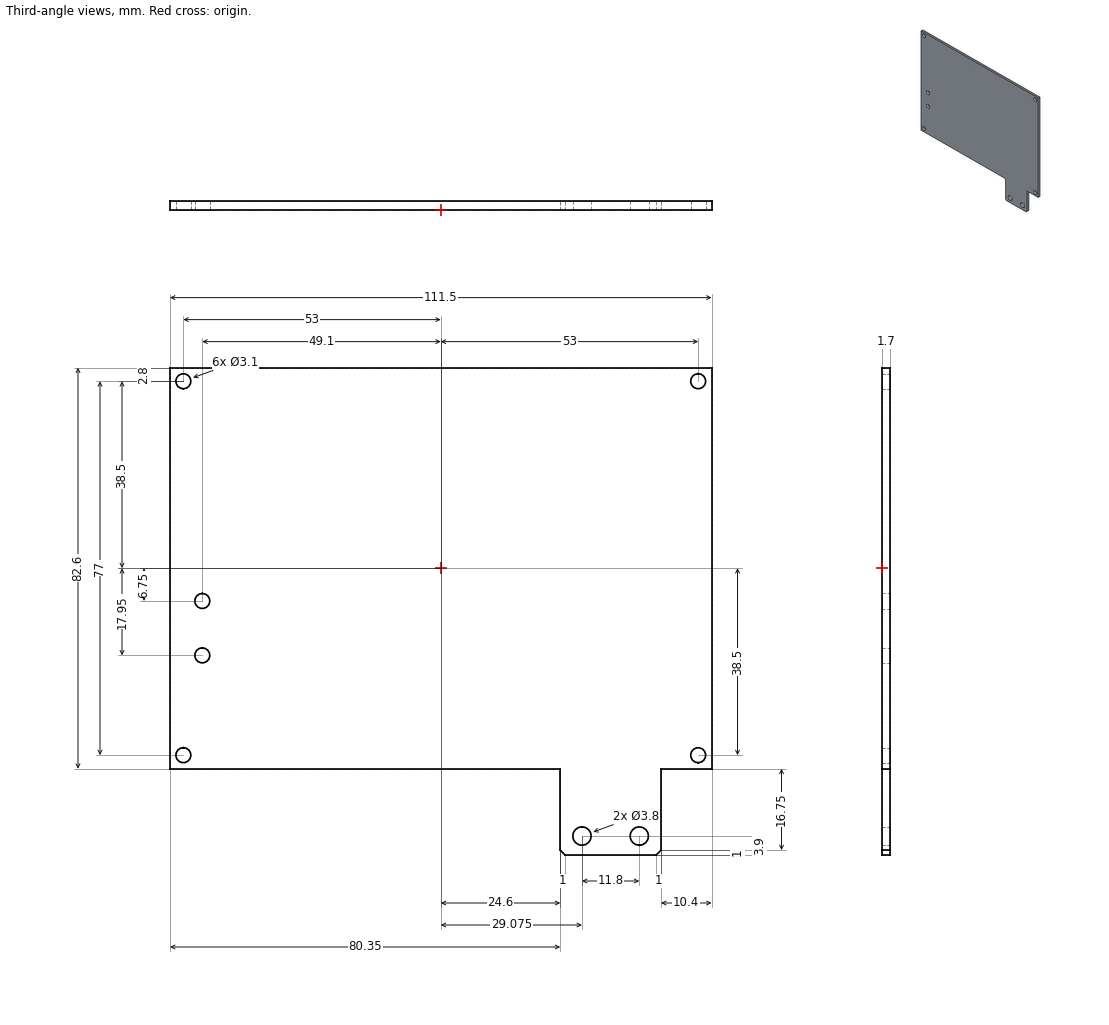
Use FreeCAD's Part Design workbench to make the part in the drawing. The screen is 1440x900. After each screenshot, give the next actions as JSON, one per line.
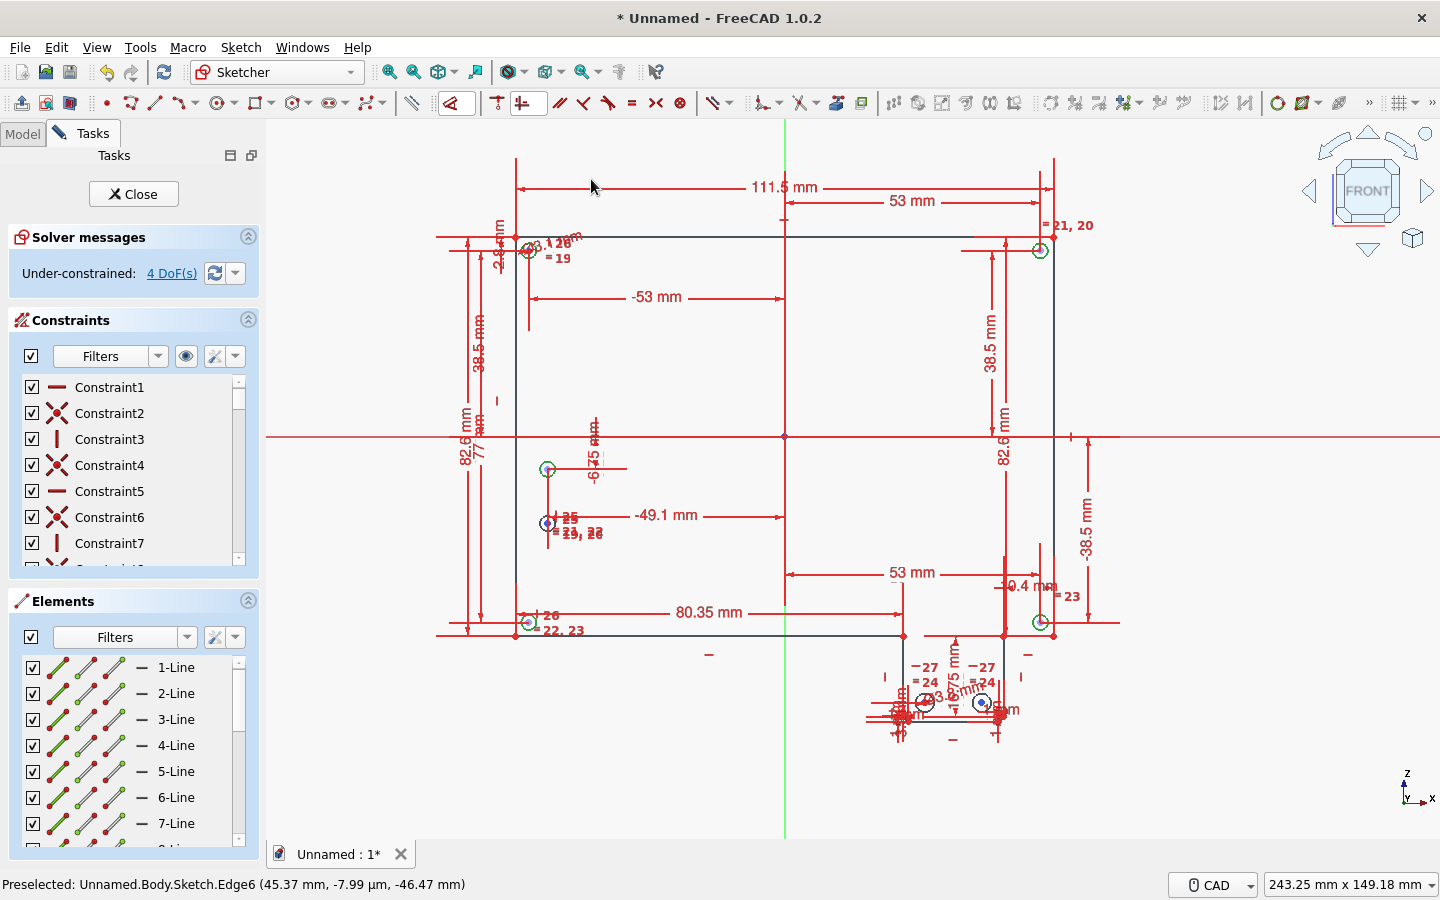
{"action": "left_click", "coordinate": [903, 636]}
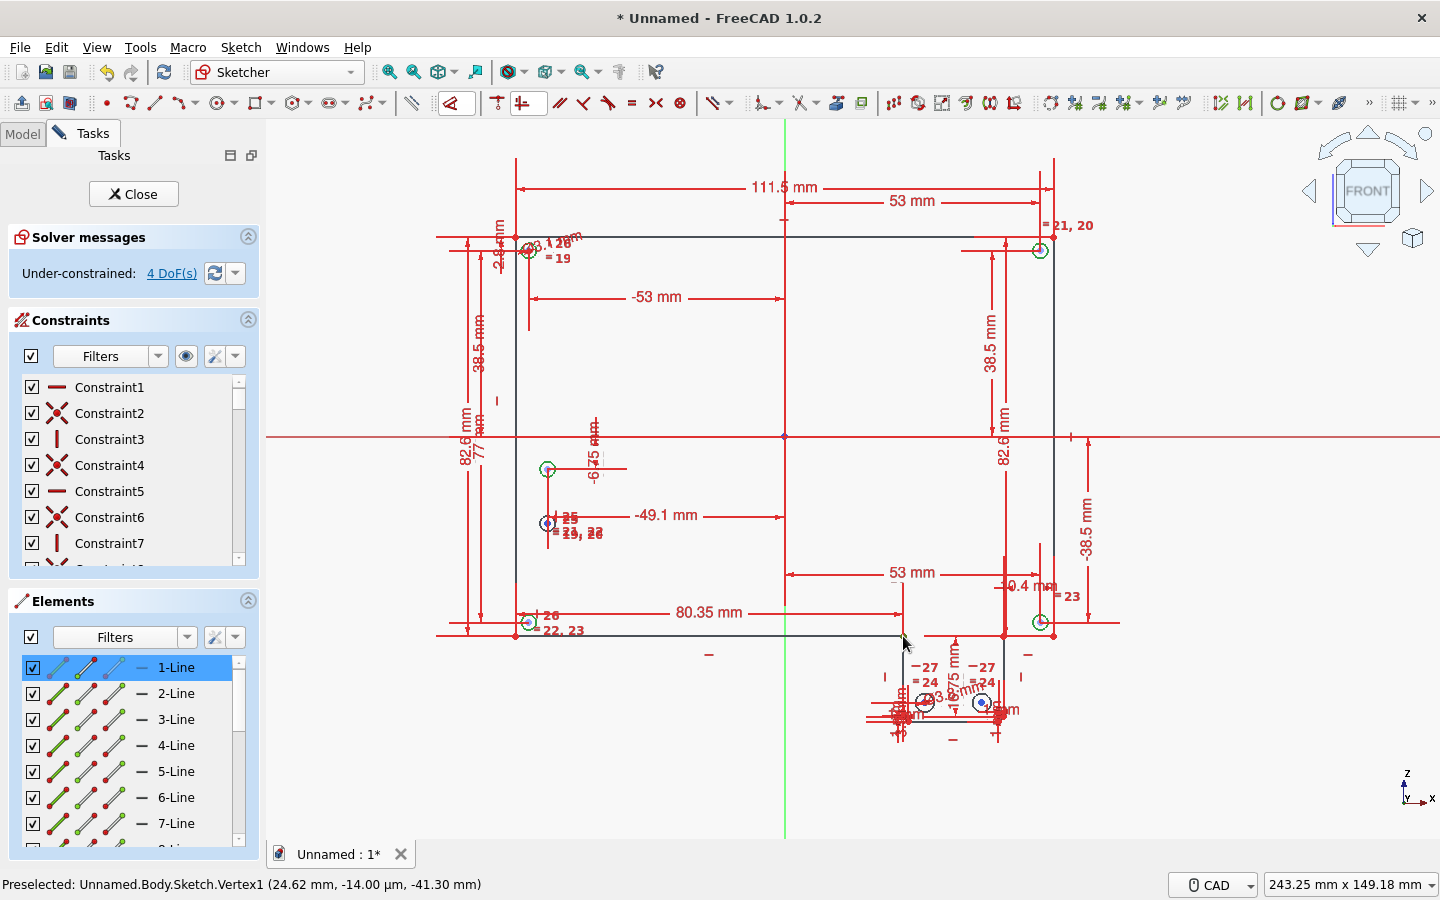
{"action": "left_click", "coordinate": [470, 104]}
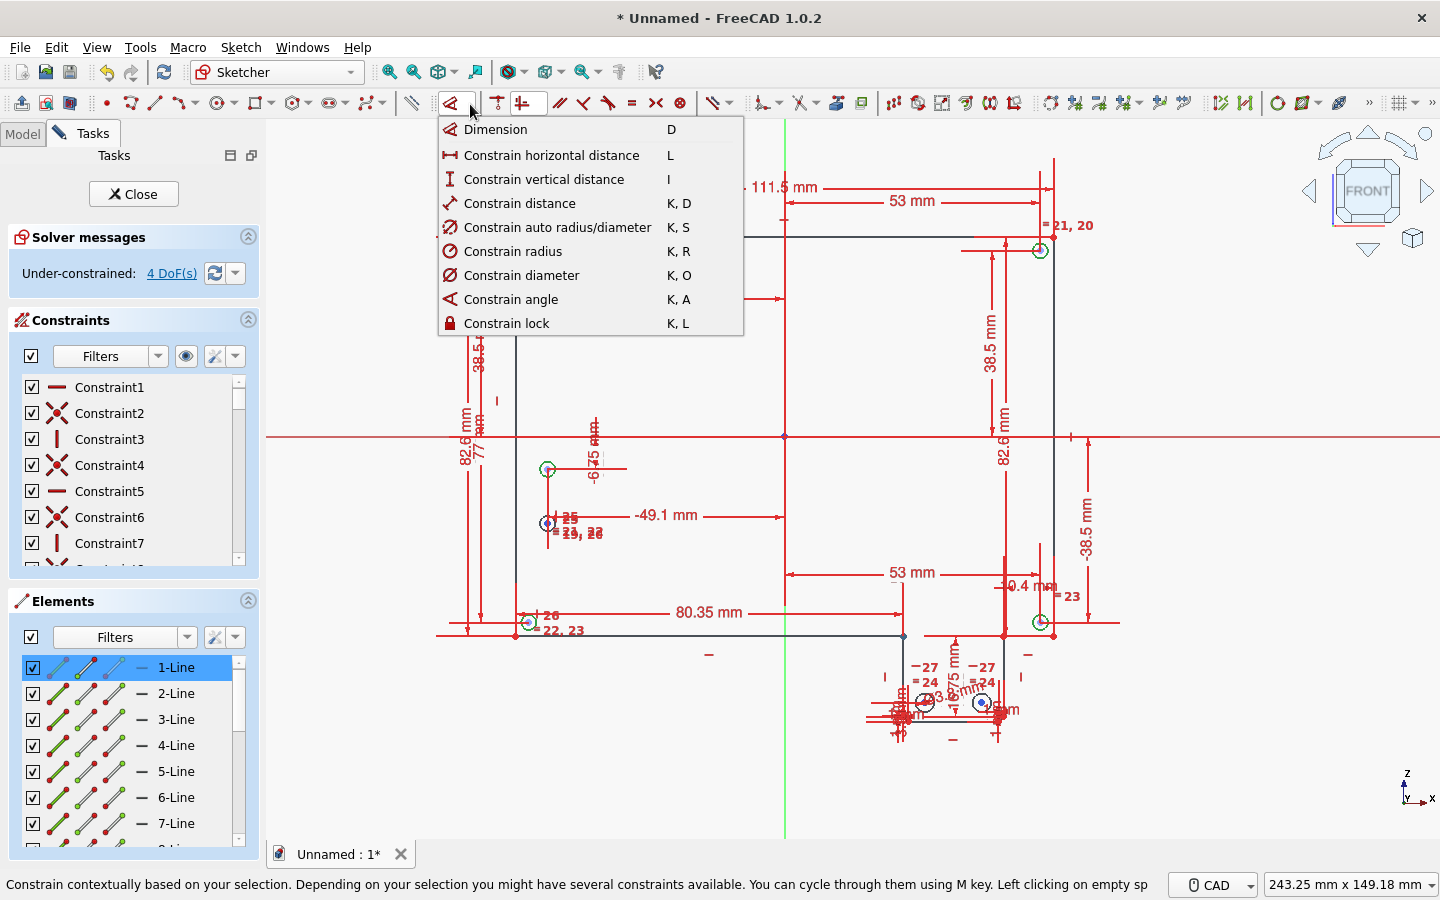
{"action": "left_click", "coordinate": [591, 155]}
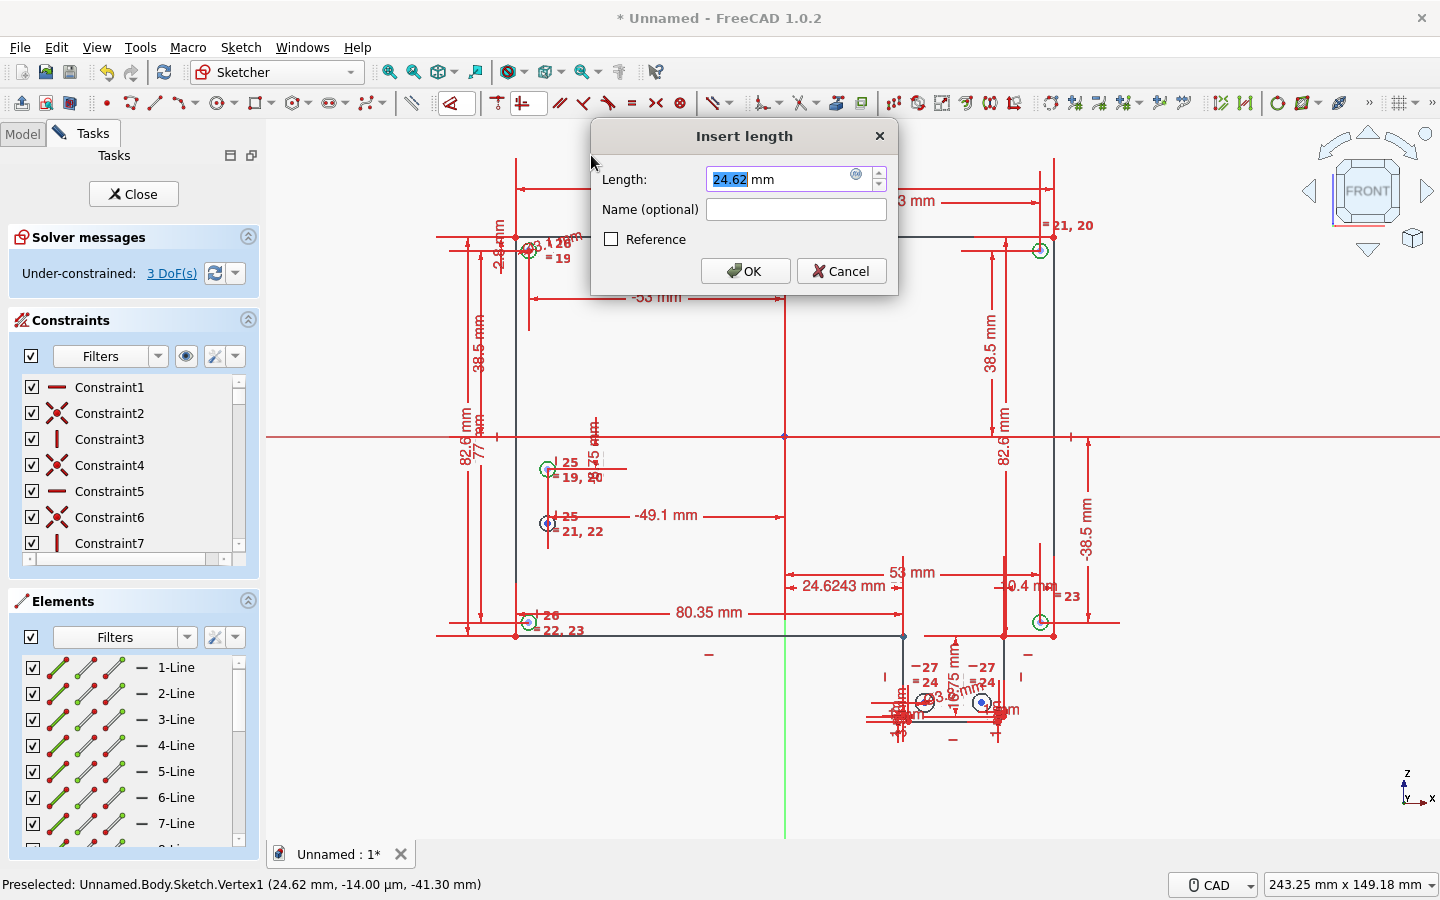
{"action": "type", "text": "24.6"}
{"action": "key", "text": "Return"}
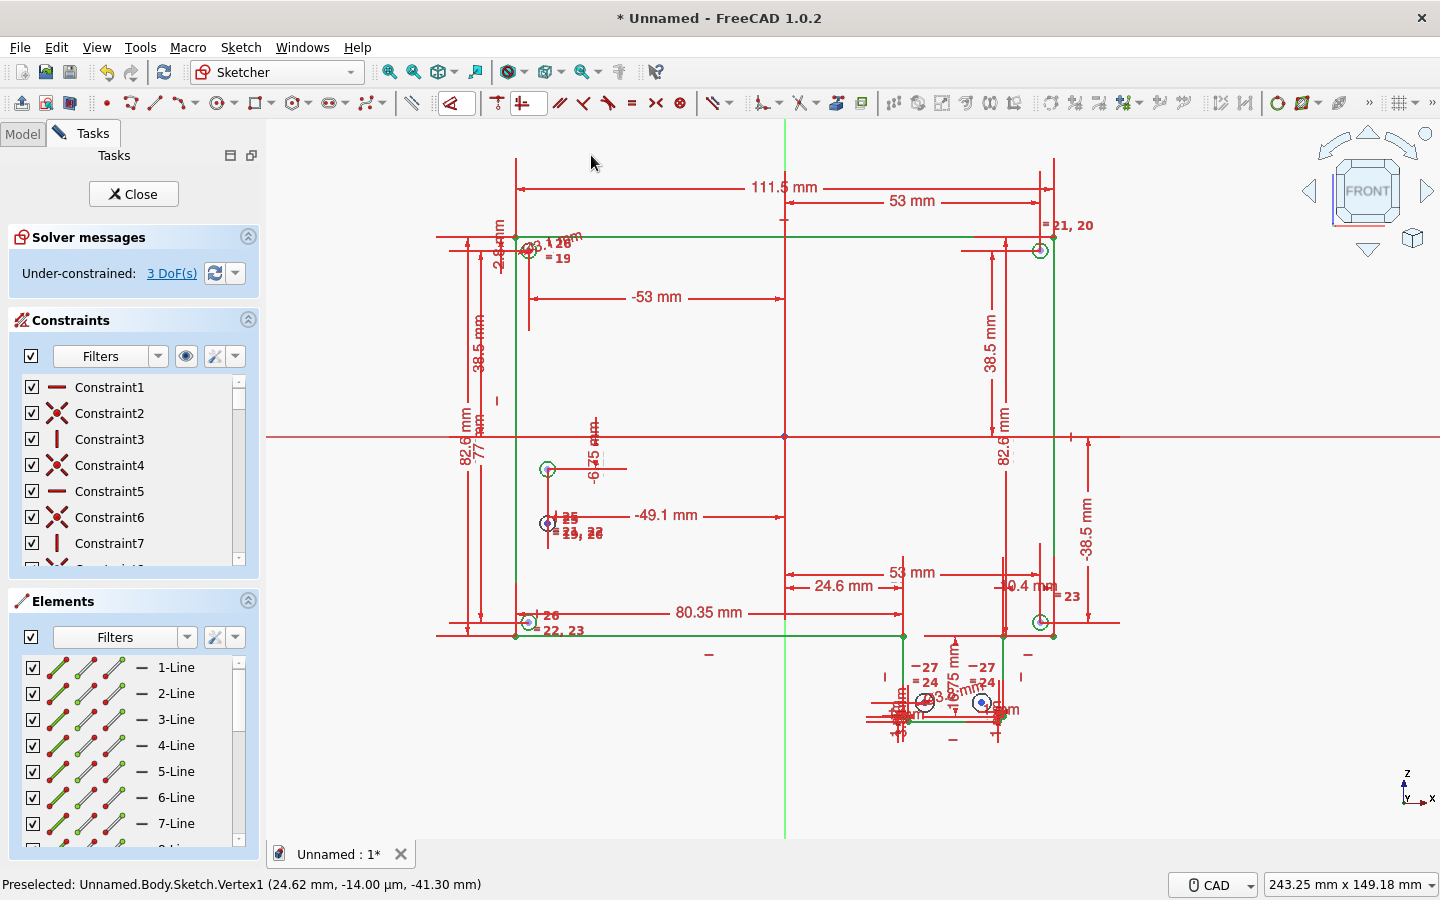
{"action": "left_click", "coordinate": [548, 524]}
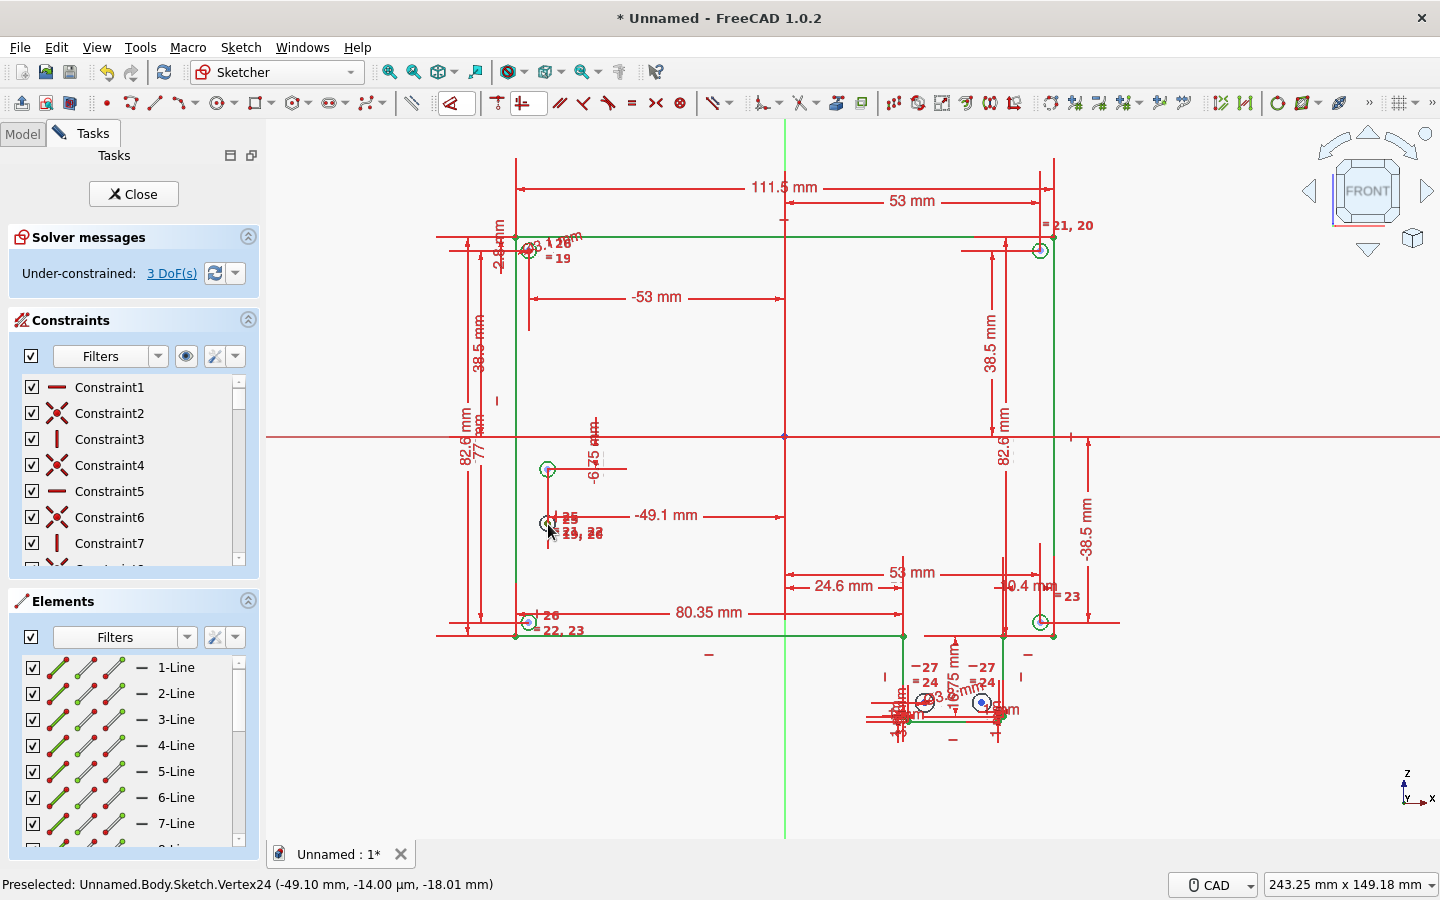
{"action": "key", "text": "i"}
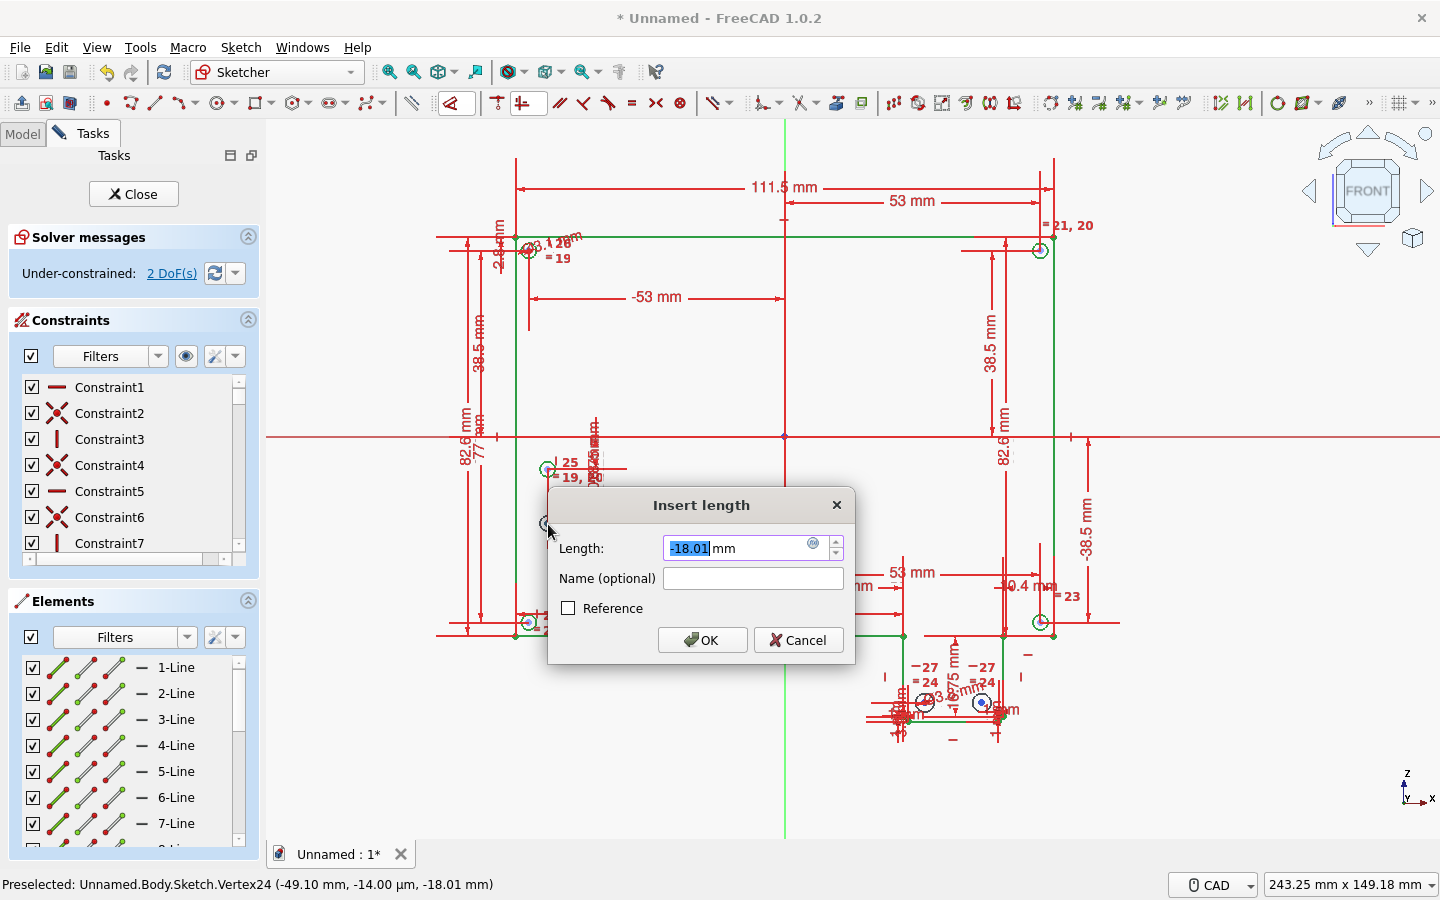
{"action": "type", "text": "-17.95"}
{"action": "key", "text": "Return"}